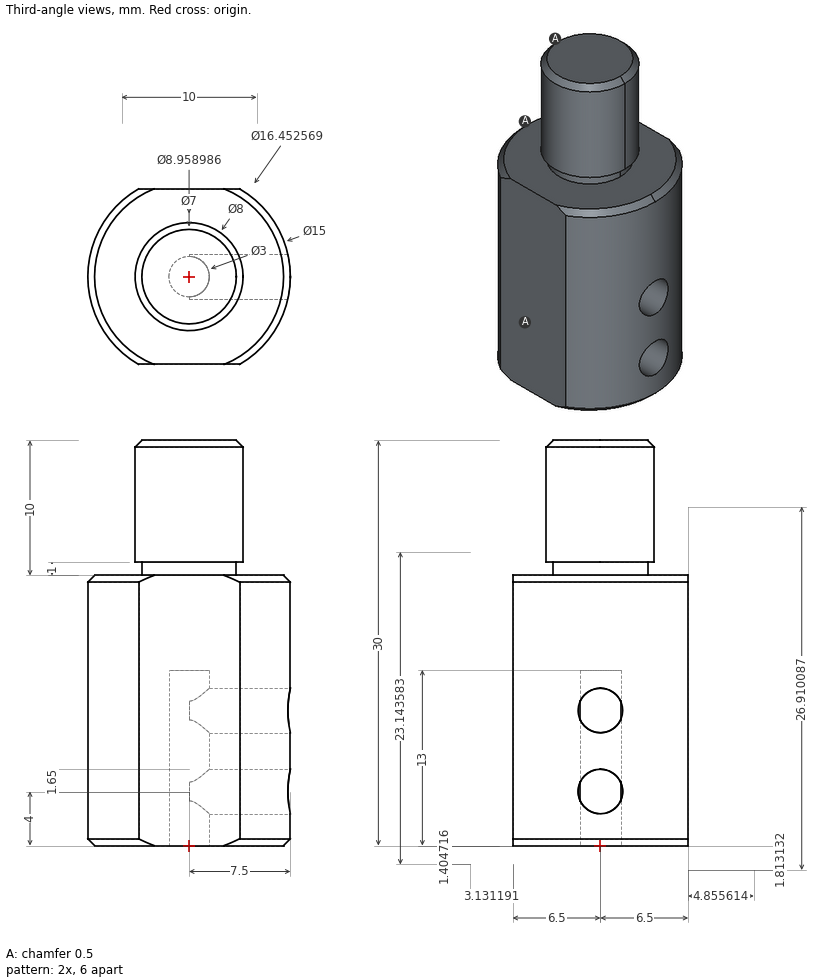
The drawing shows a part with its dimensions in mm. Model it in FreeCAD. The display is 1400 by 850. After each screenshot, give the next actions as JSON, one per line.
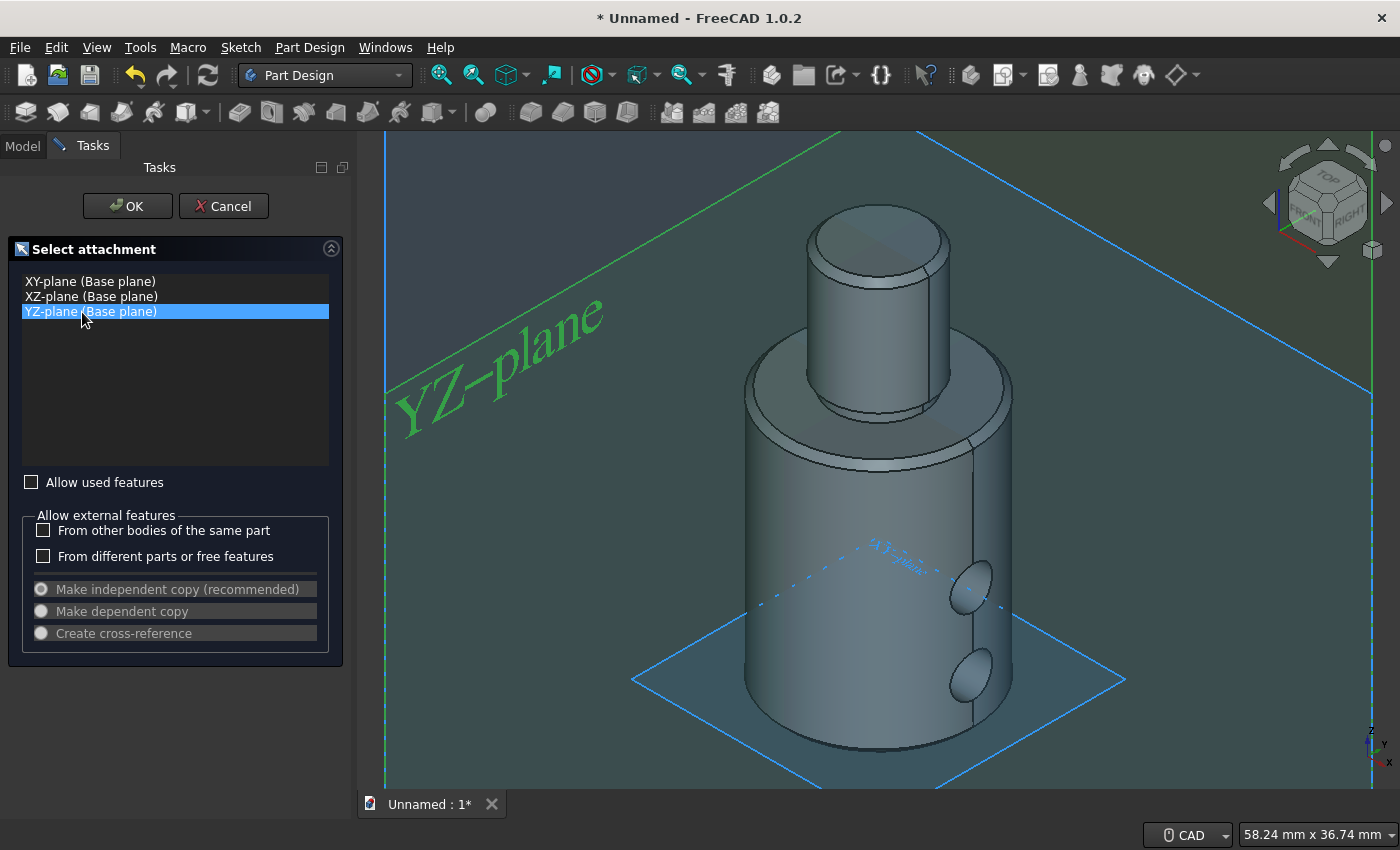
{"action": "left_click", "coordinate": [128, 206]}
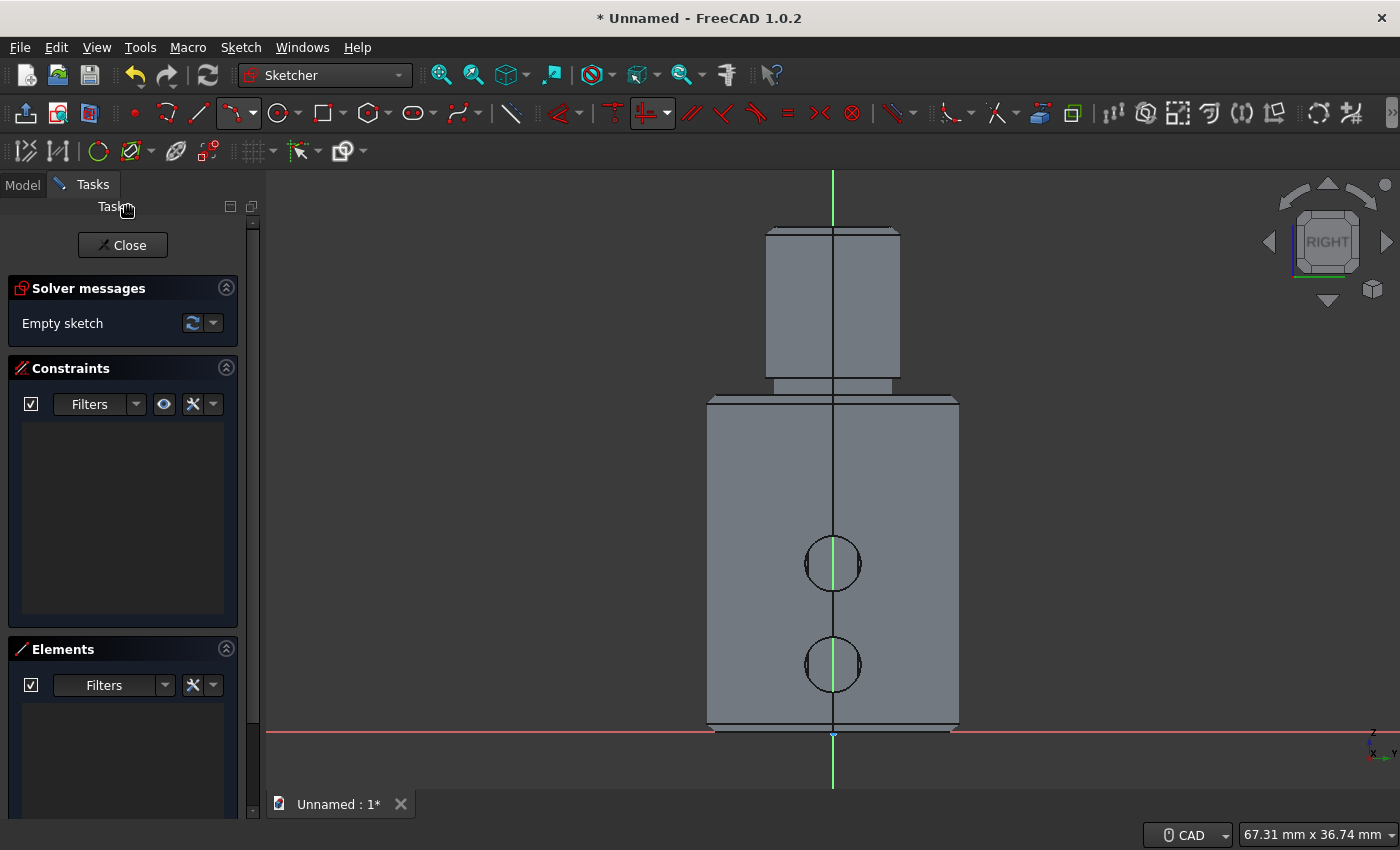
{"action": "left_click", "coordinate": [90, 114]}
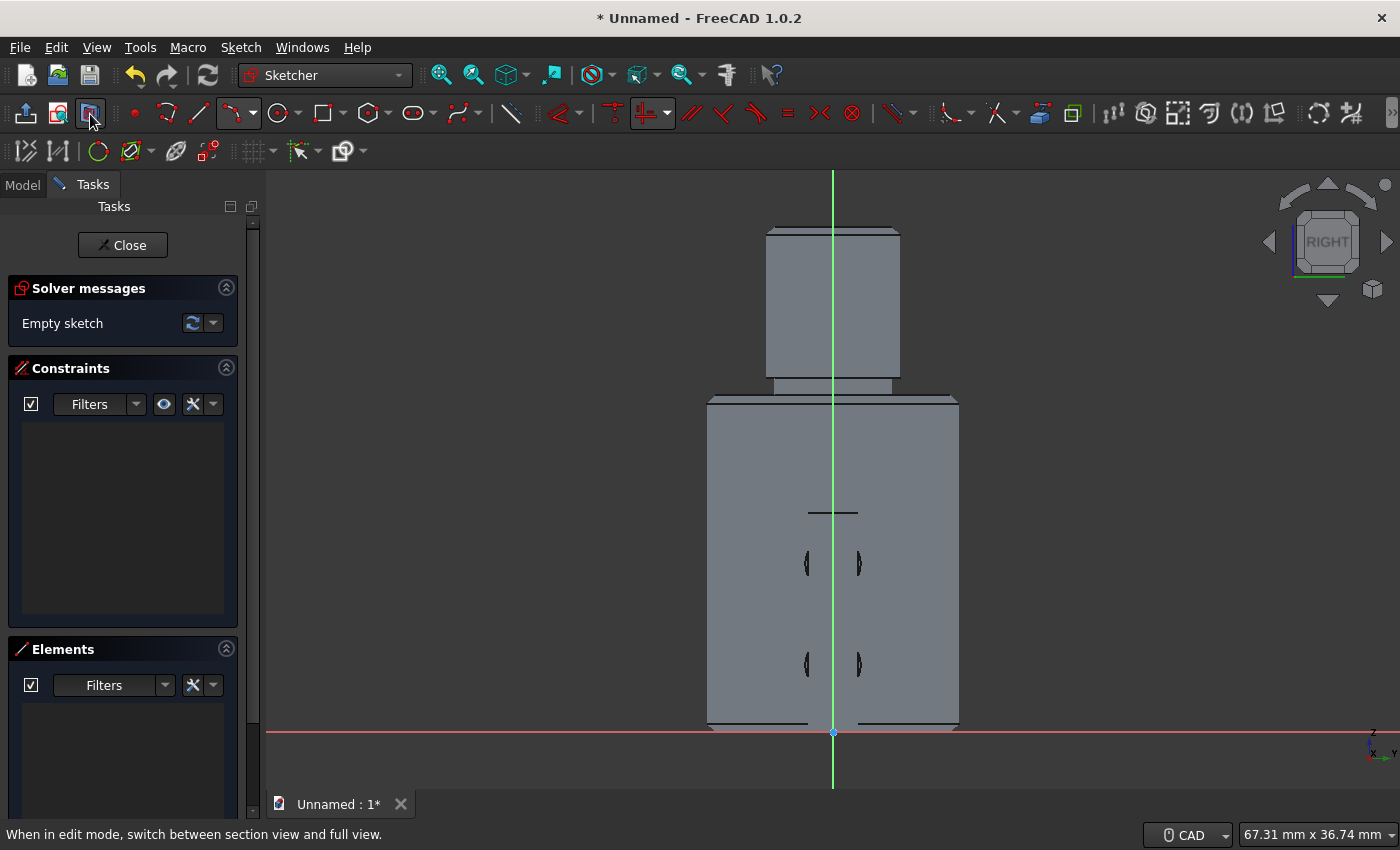
{"action": "scroll", "coordinate": [390, 224], "scroll_direction": "down", "scroll_amount": 1}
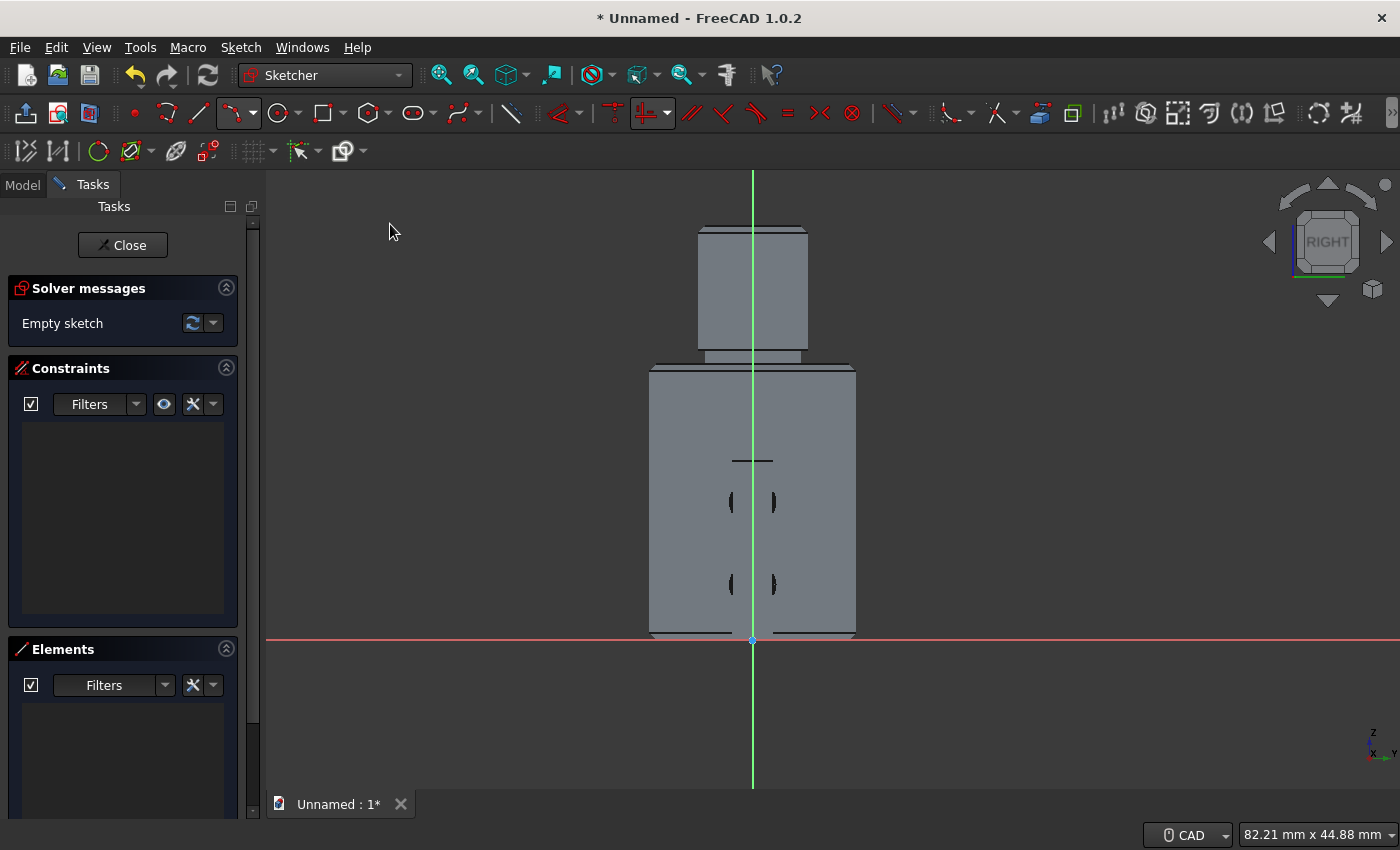
{"action": "left_click", "coordinate": [324, 114]}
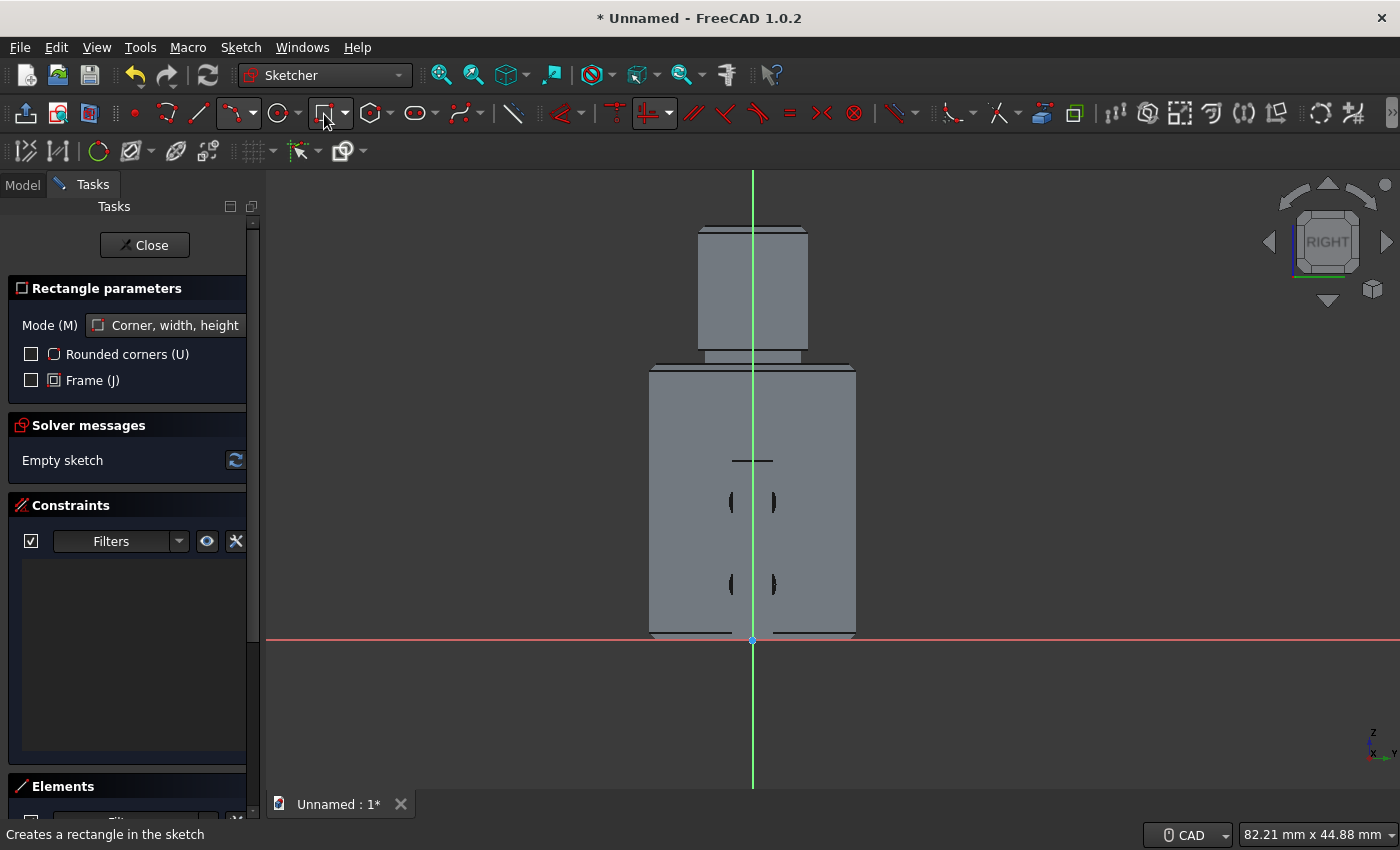
{"action": "left_click", "coordinate": [842, 294]}
{"action": "left_click", "coordinate": [909, 665]}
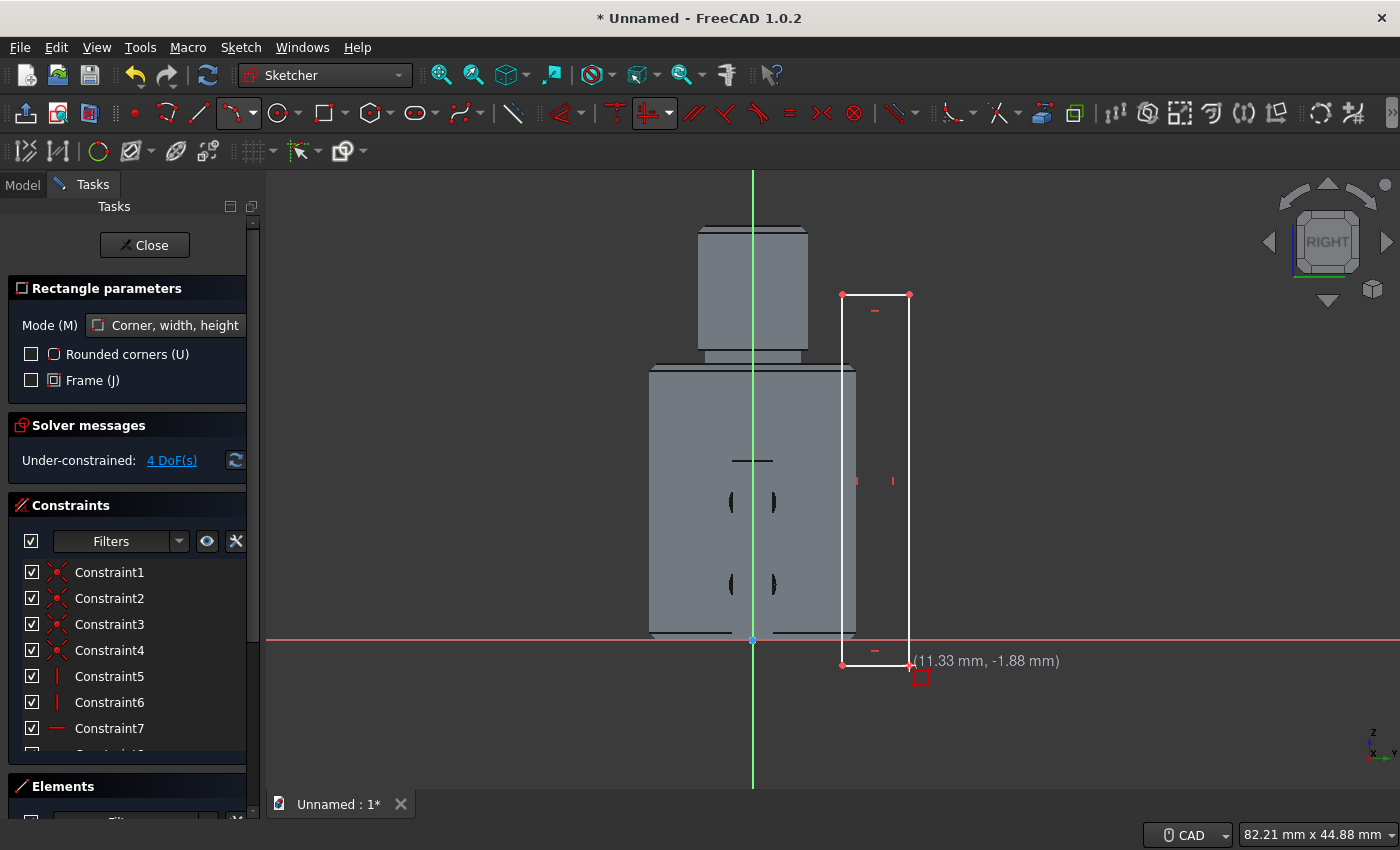
{"action": "left_click", "coordinate": [620, 340]}
{"action": "left_click", "coordinate": [663, 659]}
{"action": "key", "text": "Escape"}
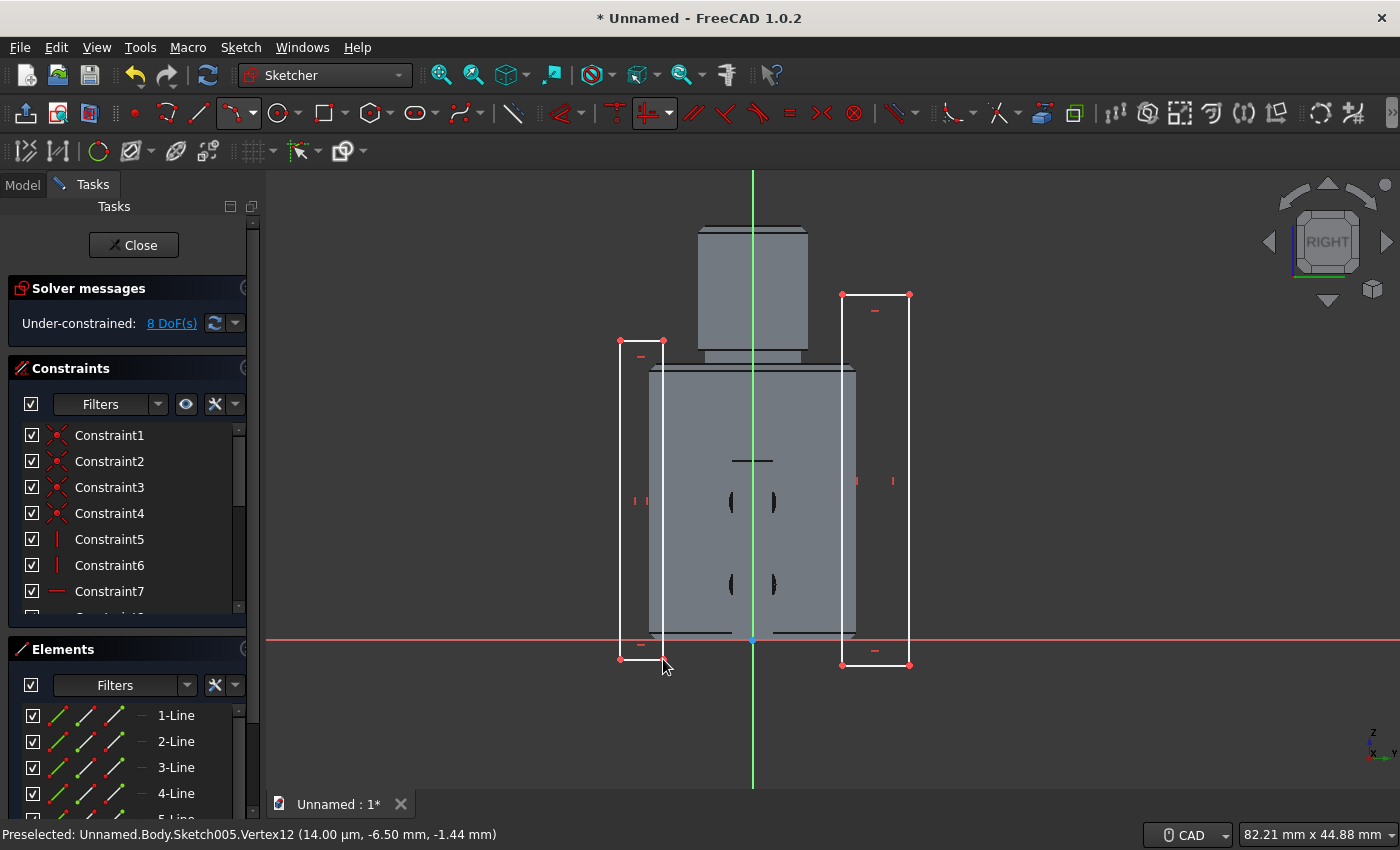
{"action": "left_click", "coordinate": [560, 114]}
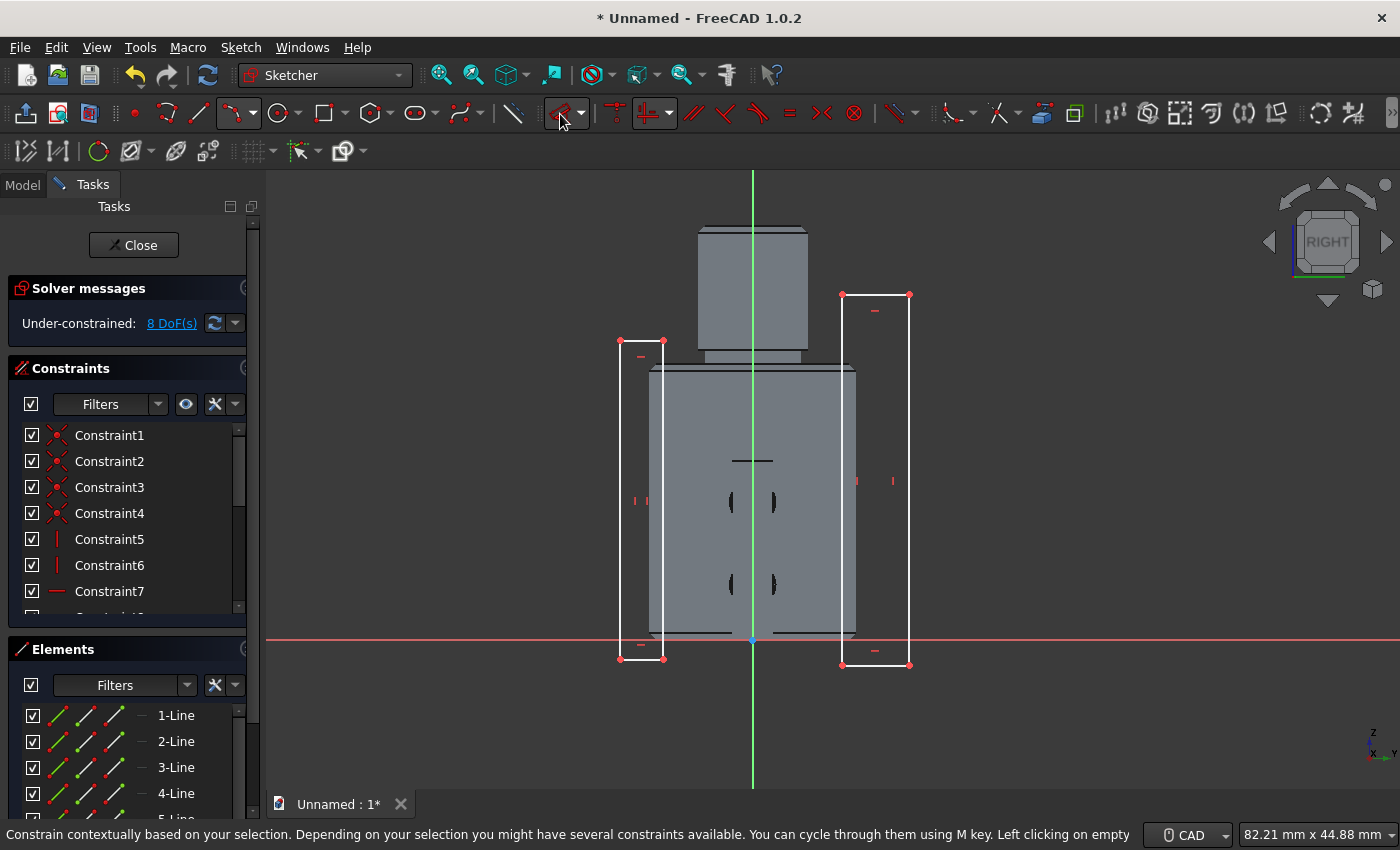
{"action": "left_click", "coordinate": [842, 295]}
{"action": "left_click", "coordinate": [797, 261]}